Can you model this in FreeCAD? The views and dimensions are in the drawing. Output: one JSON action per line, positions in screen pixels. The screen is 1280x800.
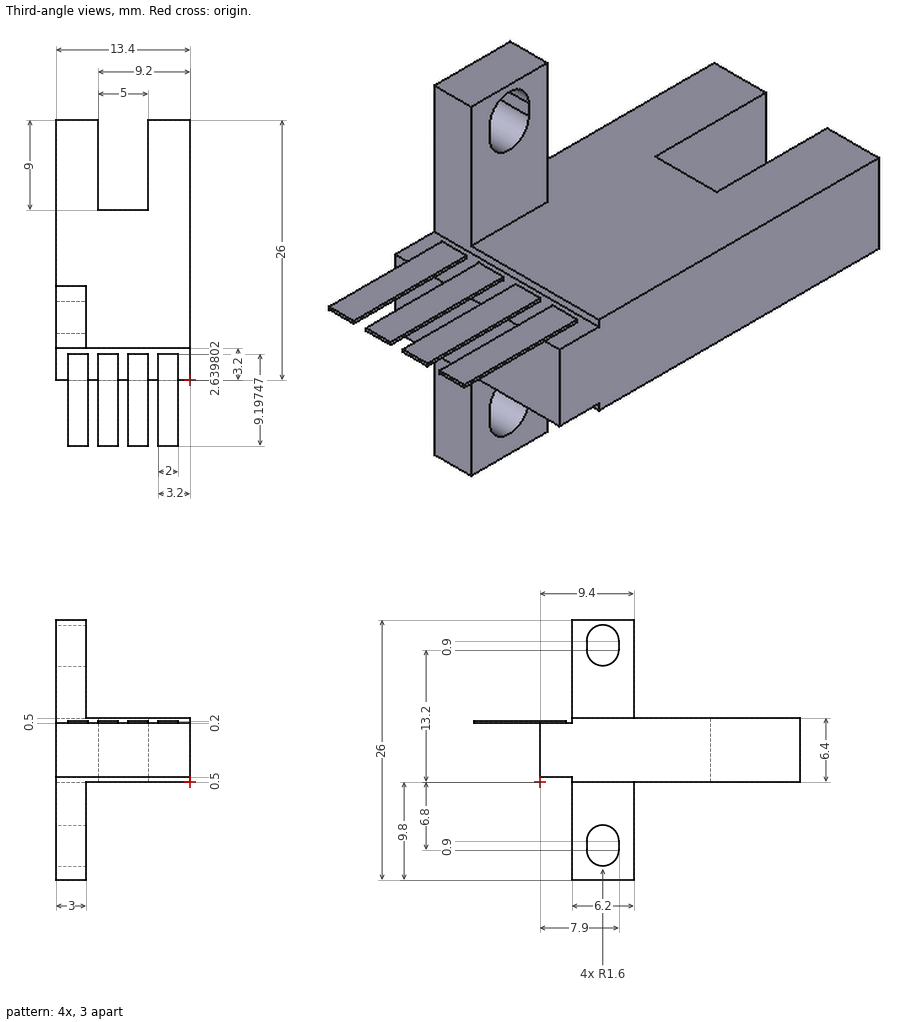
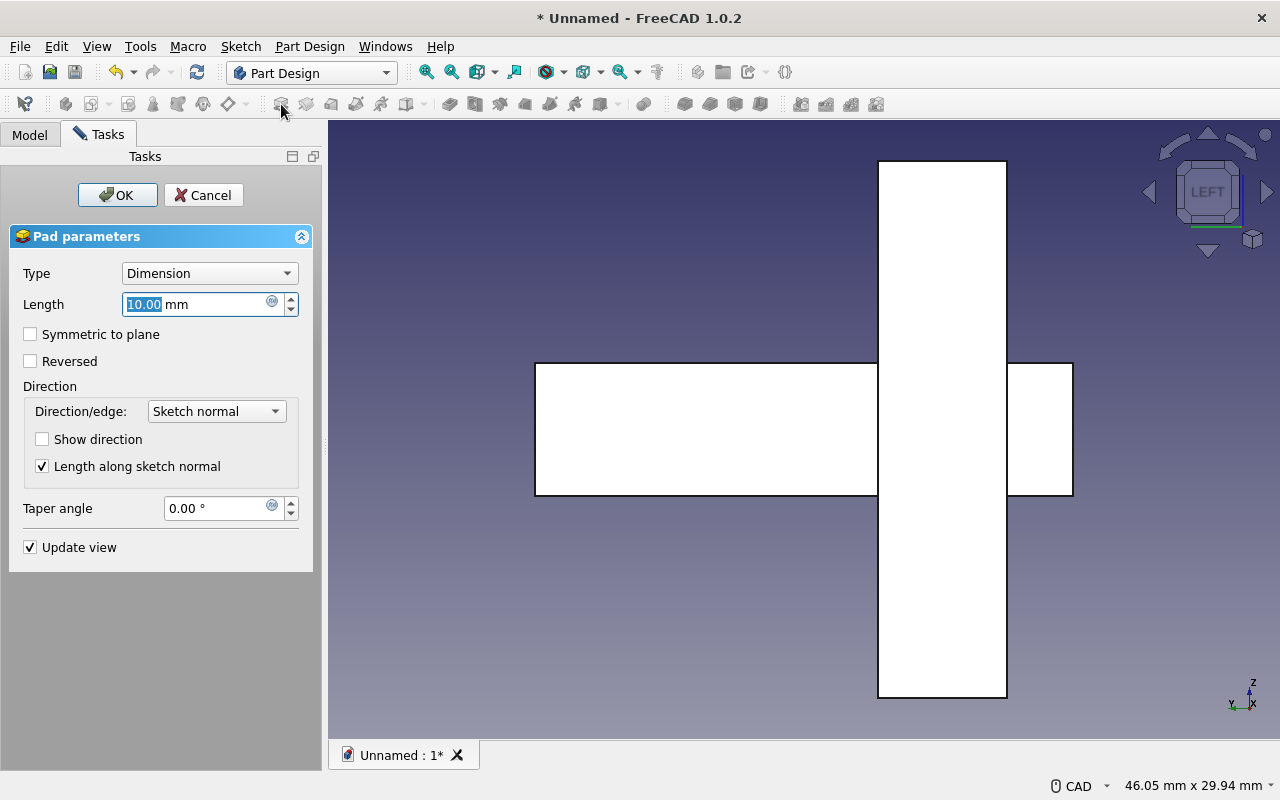
{"action": "type", "text": "3"}
{"action": "key", "text": "Tab"}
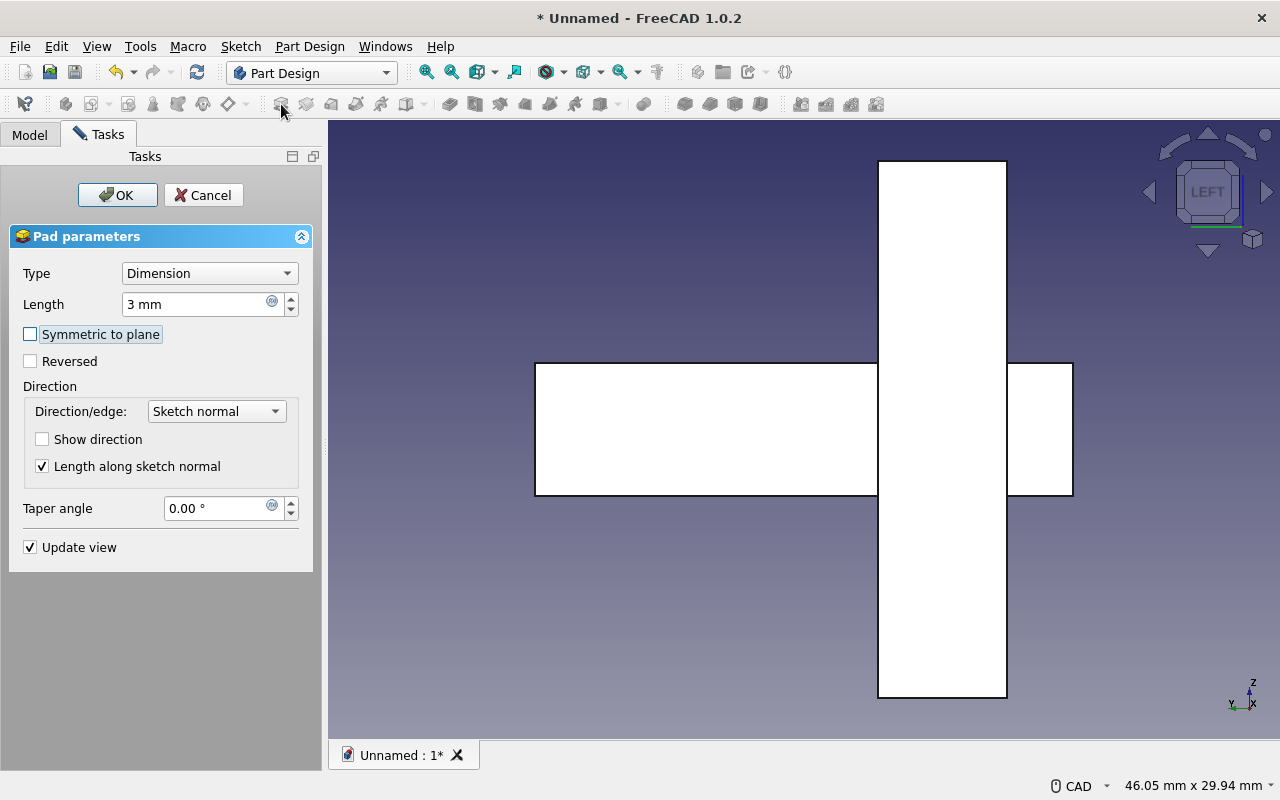
{"action": "left_click", "coordinate": [31, 361]}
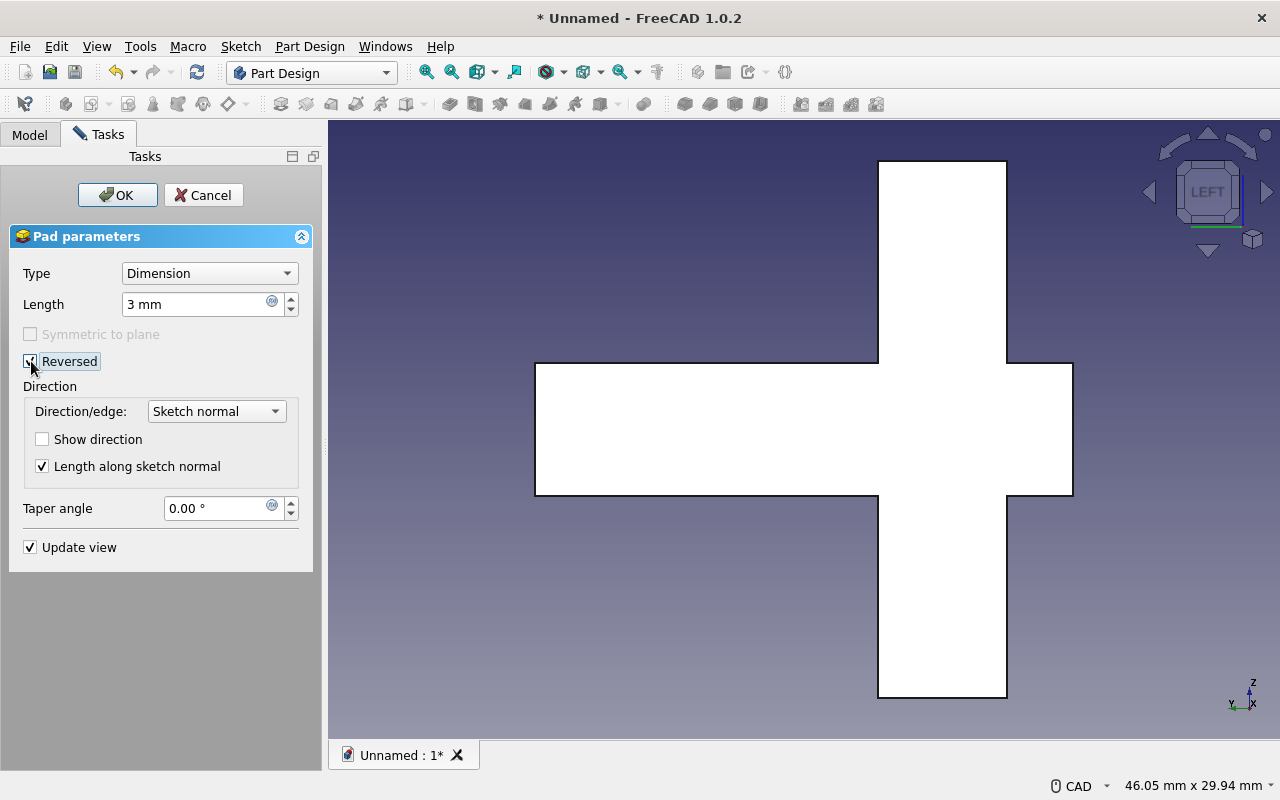
{"action": "left_click", "coordinate": [118, 195]}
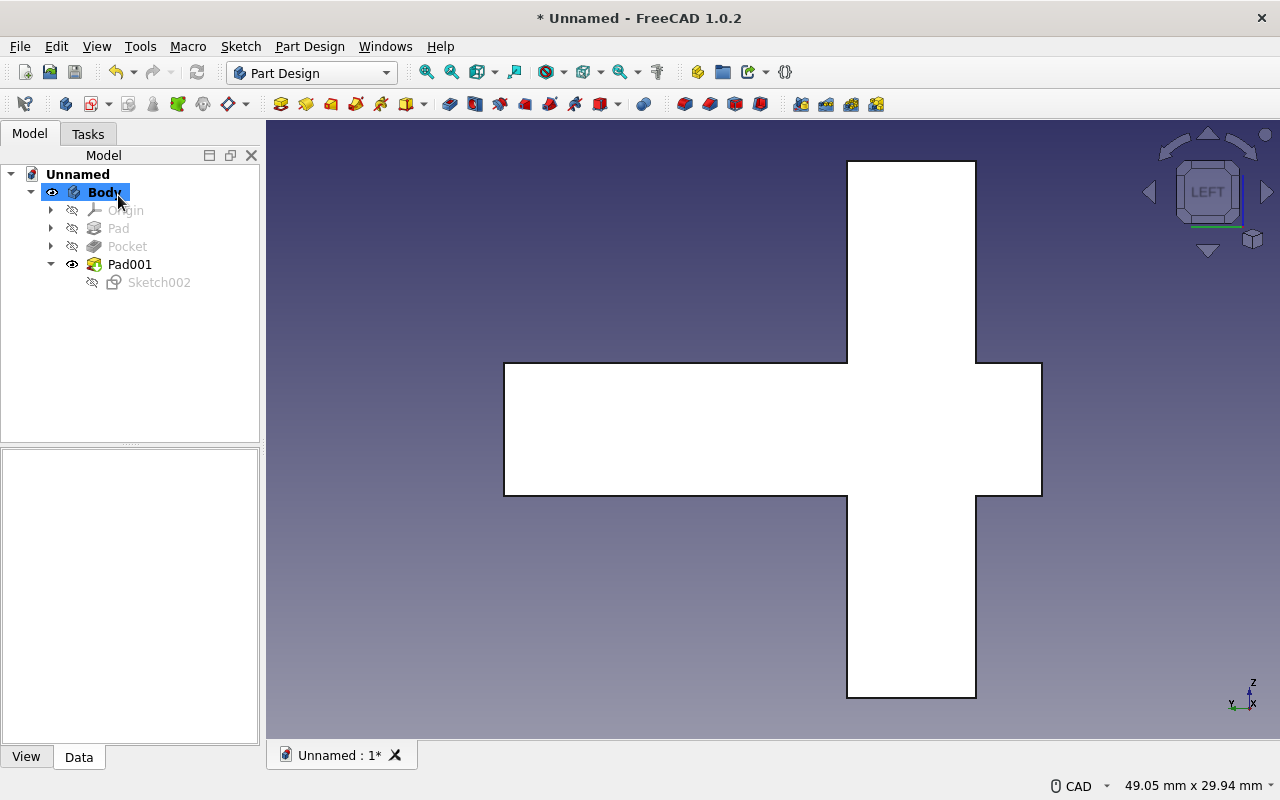
{"action": "left_click", "coordinate": [927, 428]}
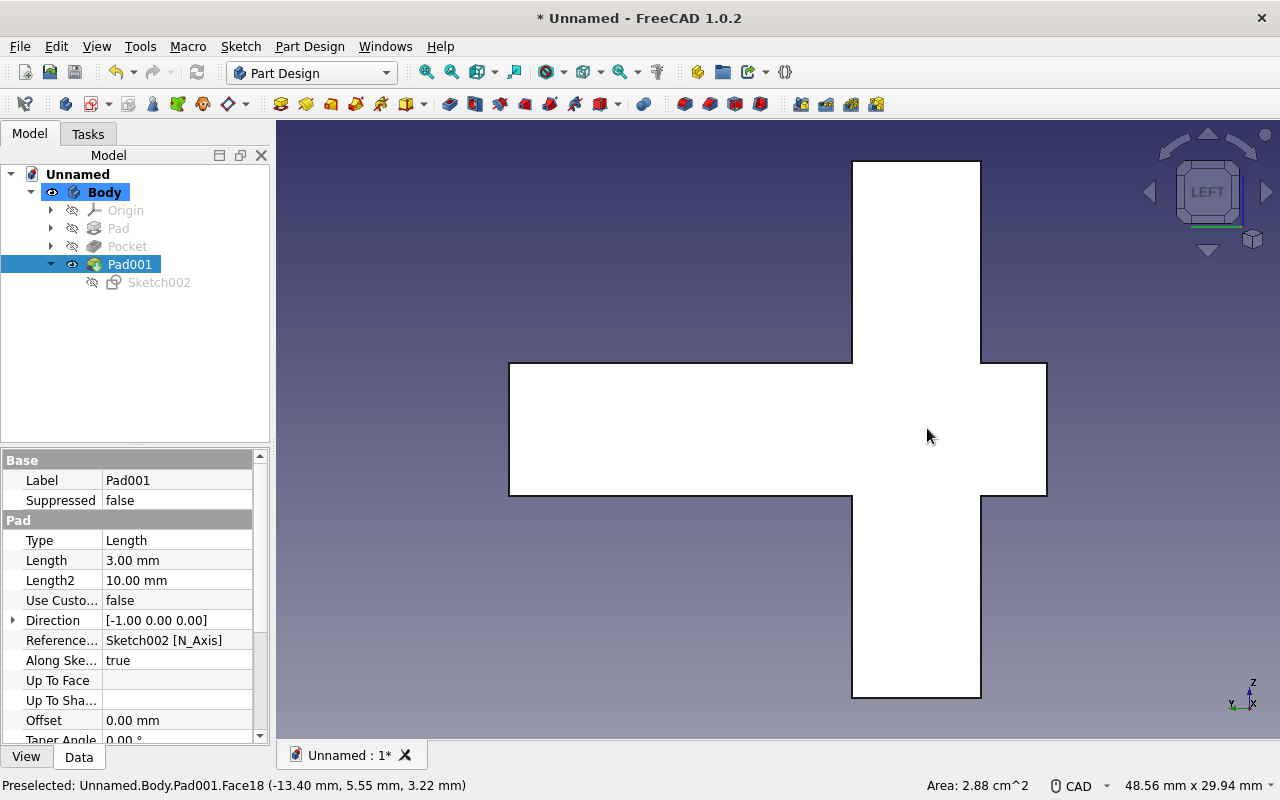
{"action": "left_click", "coordinate": [90, 104]}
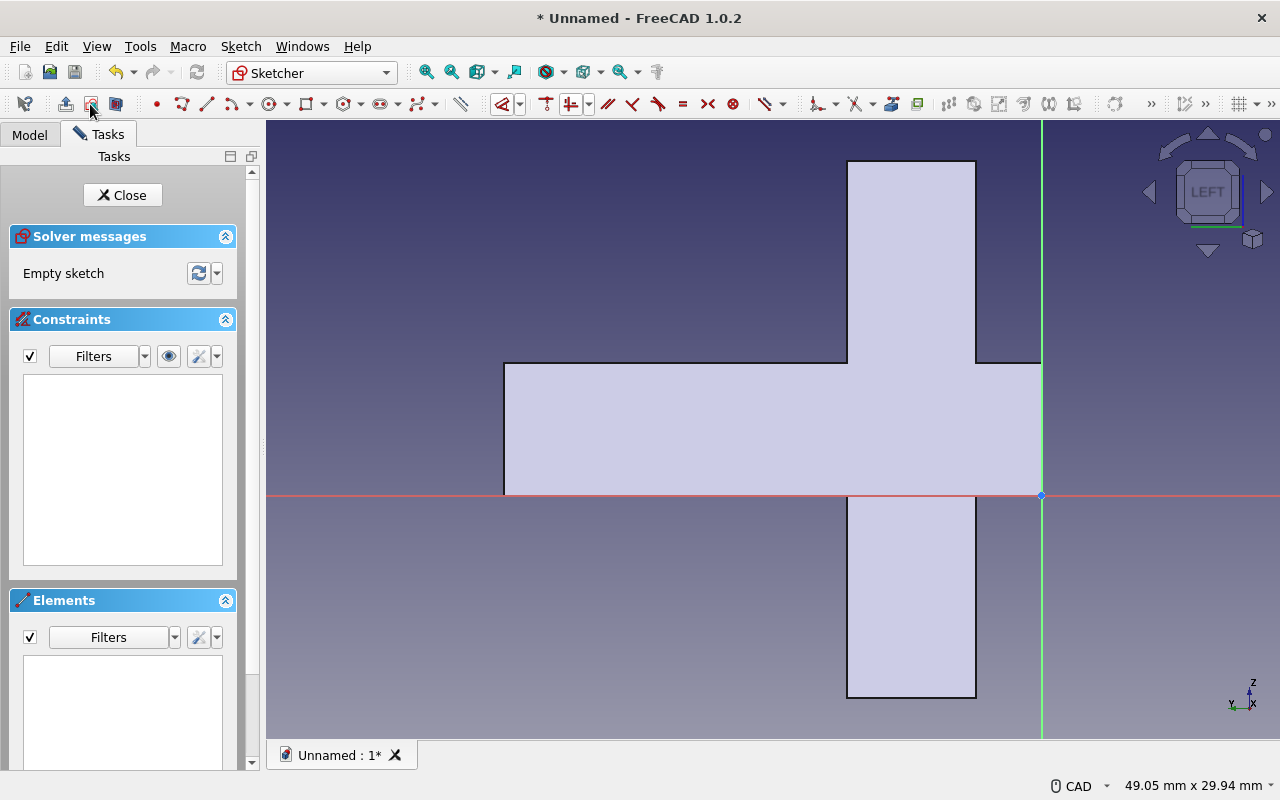
{"action": "scroll", "coordinate": [294, 472], "scroll_direction": "down", "scroll_amount": 1}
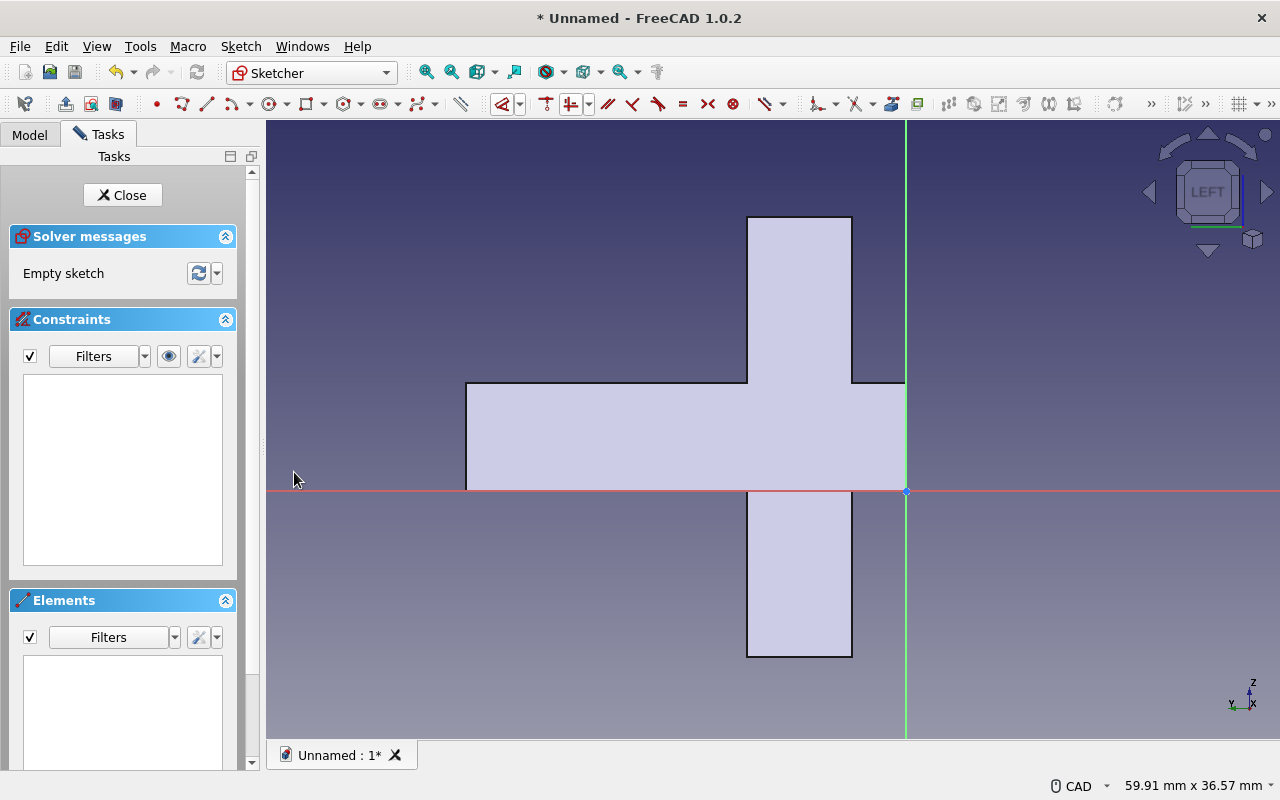
{"action": "key", "text": "g s"}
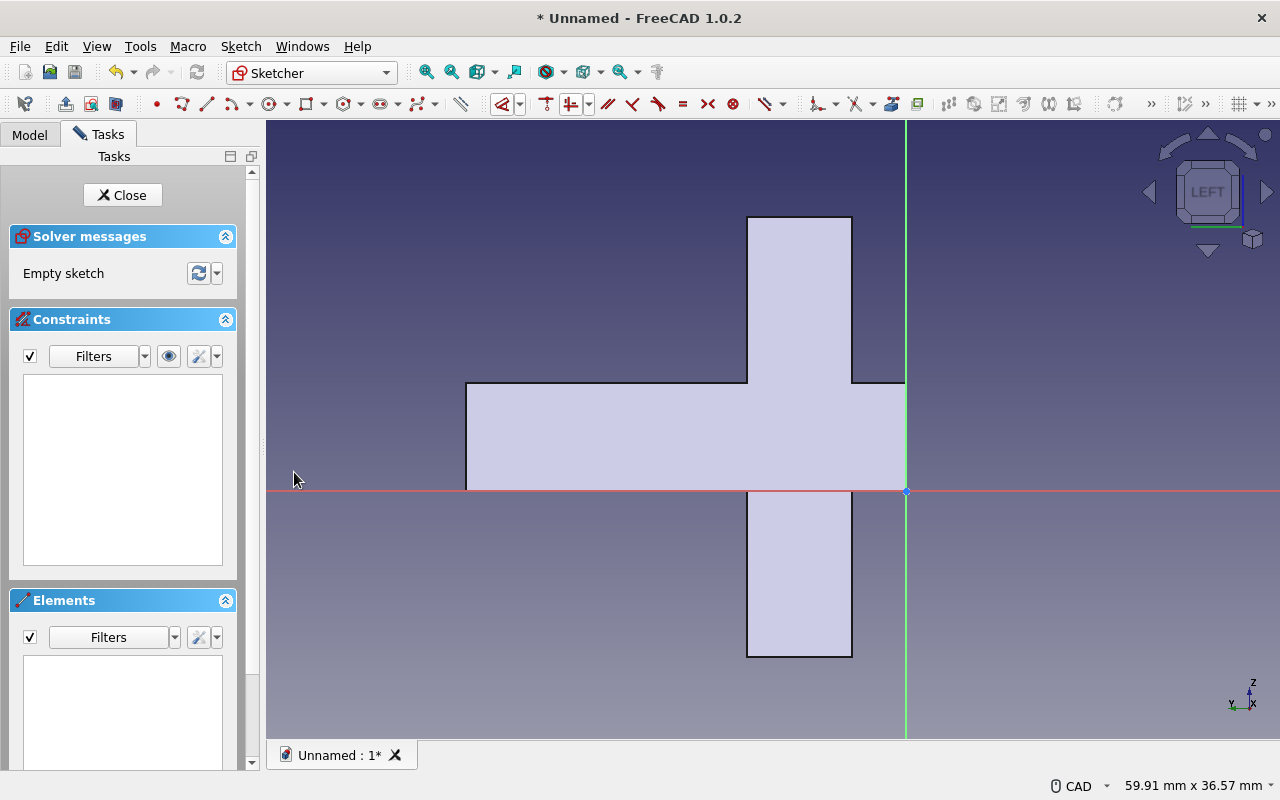
{"action": "left_click", "coordinate": [800, 607]}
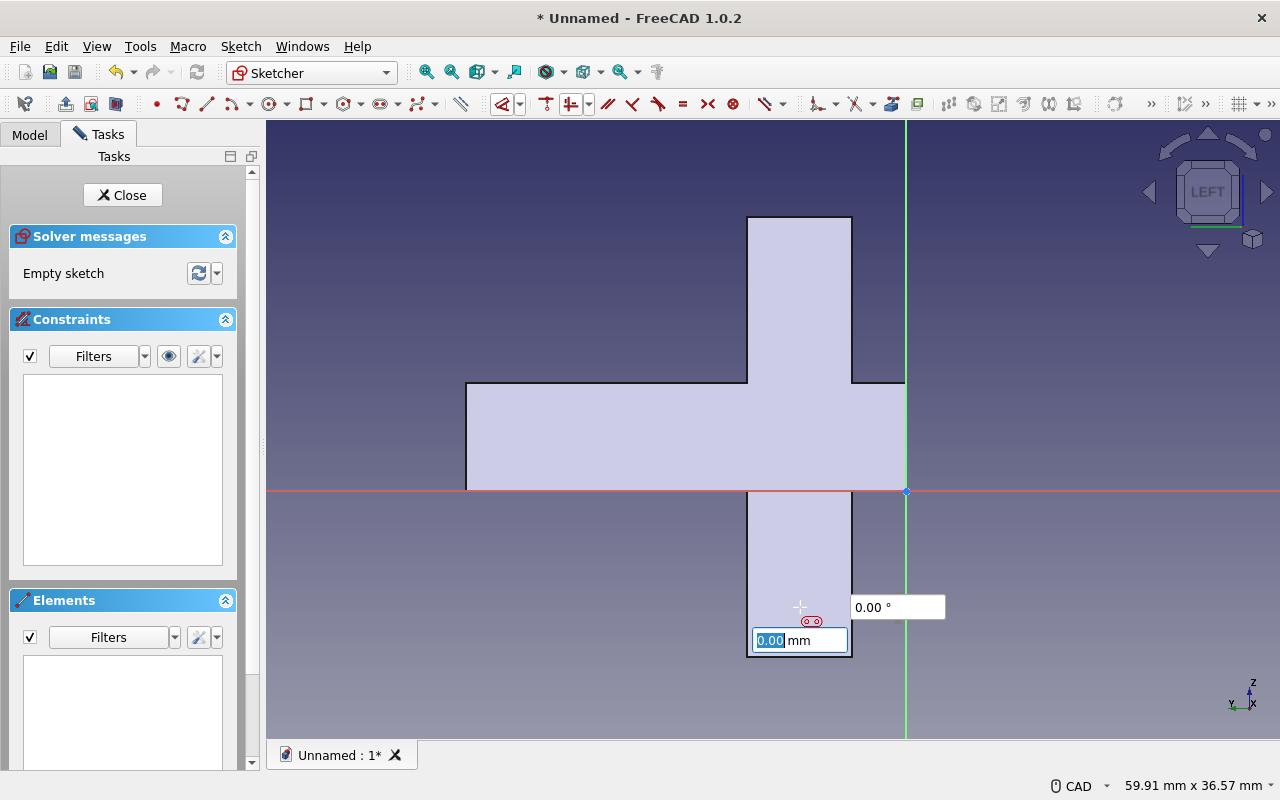
{"action": "left_click", "coordinate": [800, 591]}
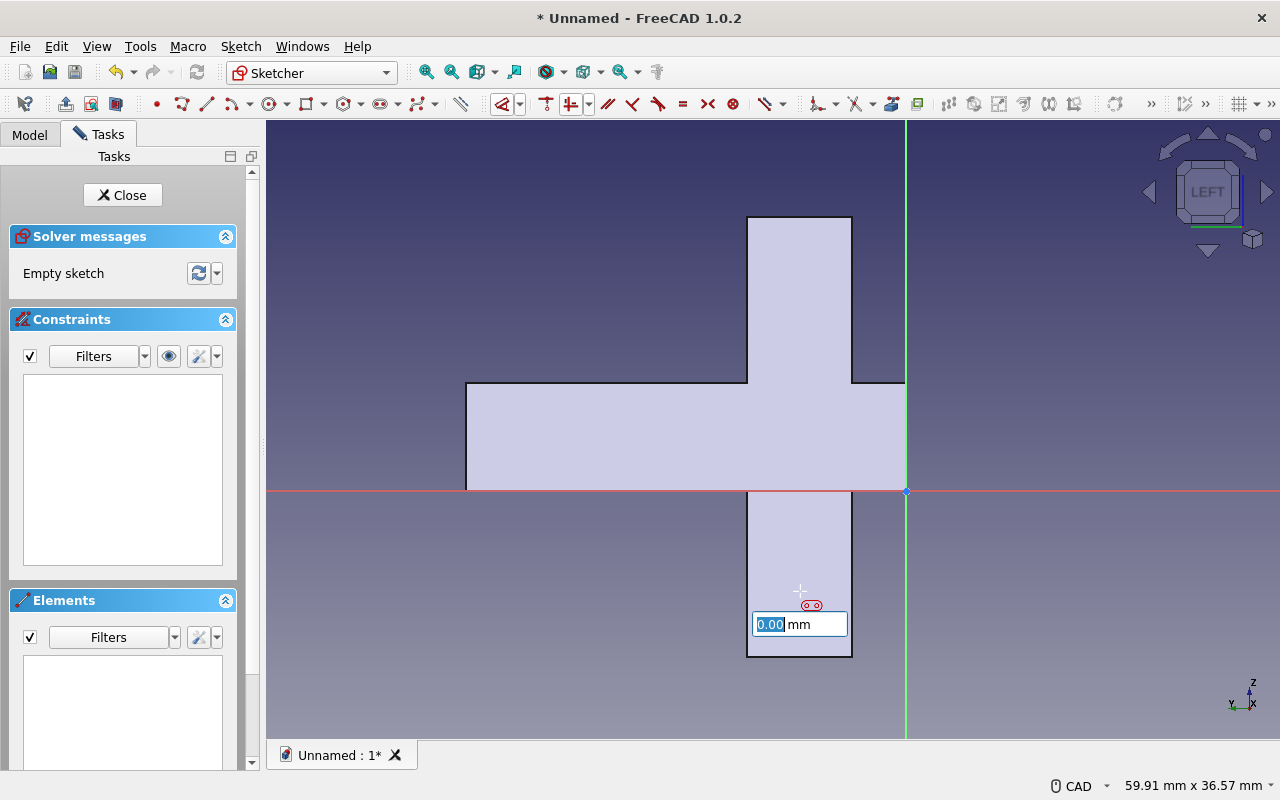
{"action": "left_click", "coordinate": [772, 599]}